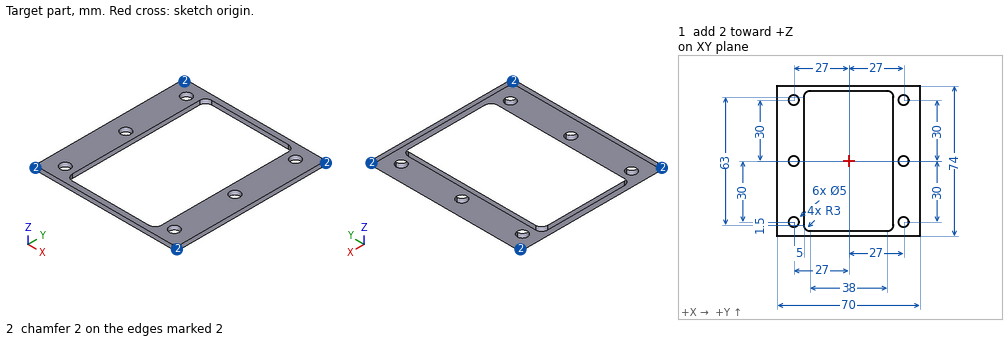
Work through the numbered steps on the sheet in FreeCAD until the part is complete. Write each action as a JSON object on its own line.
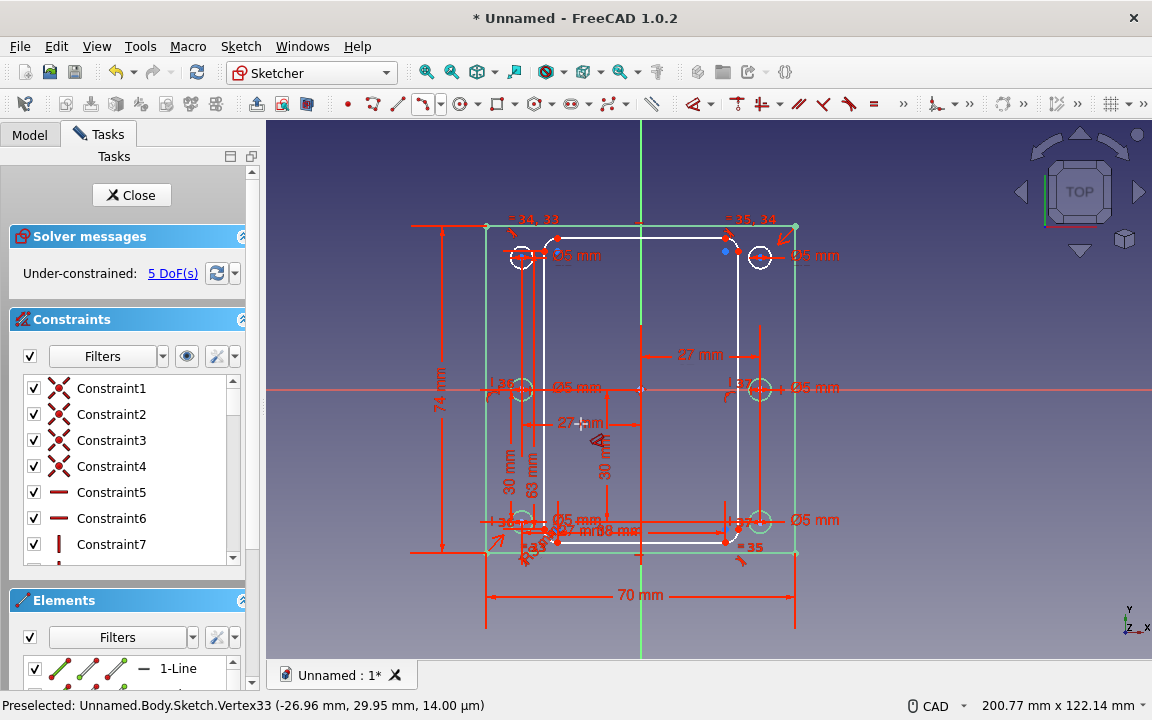
{"action": "left_click", "coordinate": [522, 258]}
{"action": "left_click", "coordinate": [675, 324]}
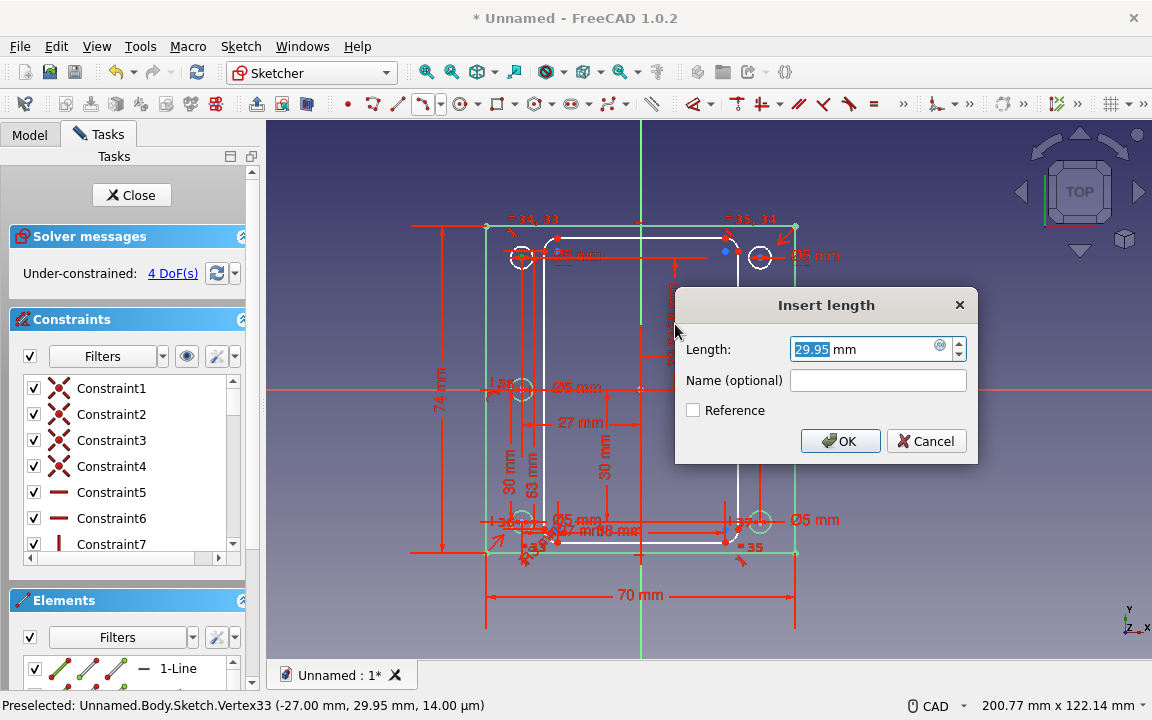
{"action": "type", "text": "30"}
{"action": "key", "text": "Return"}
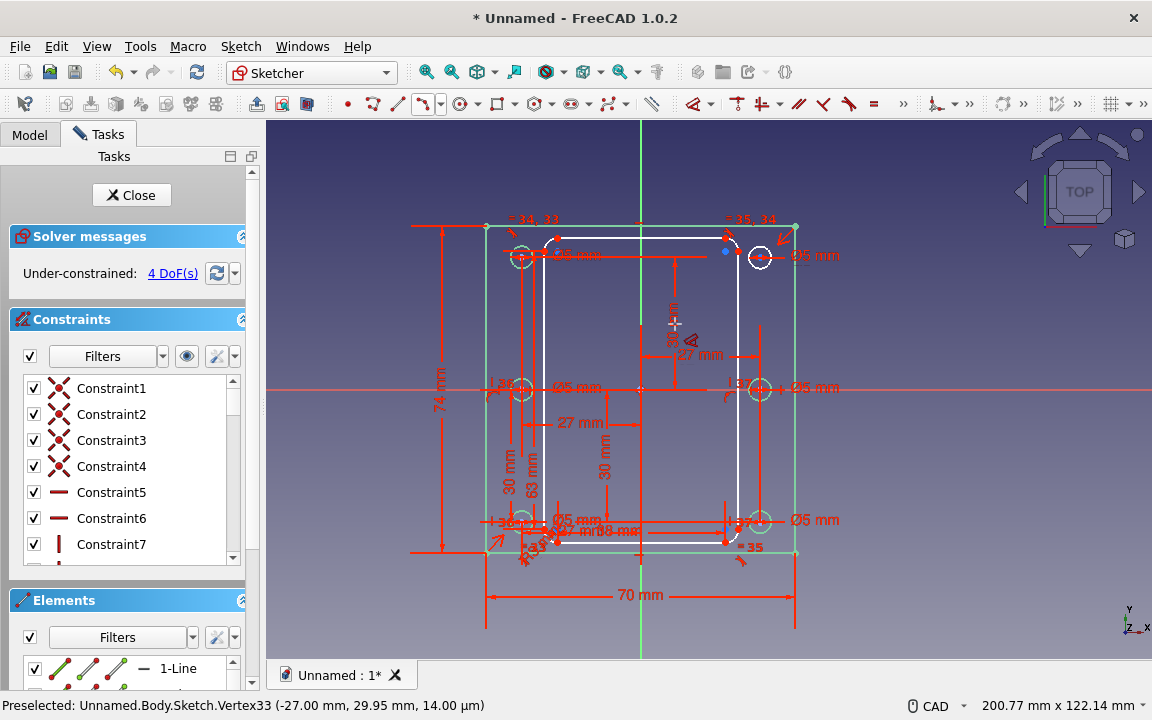
{"action": "left_click", "coordinate": [760, 258]}
{"action": "left_click", "coordinate": [701, 424]}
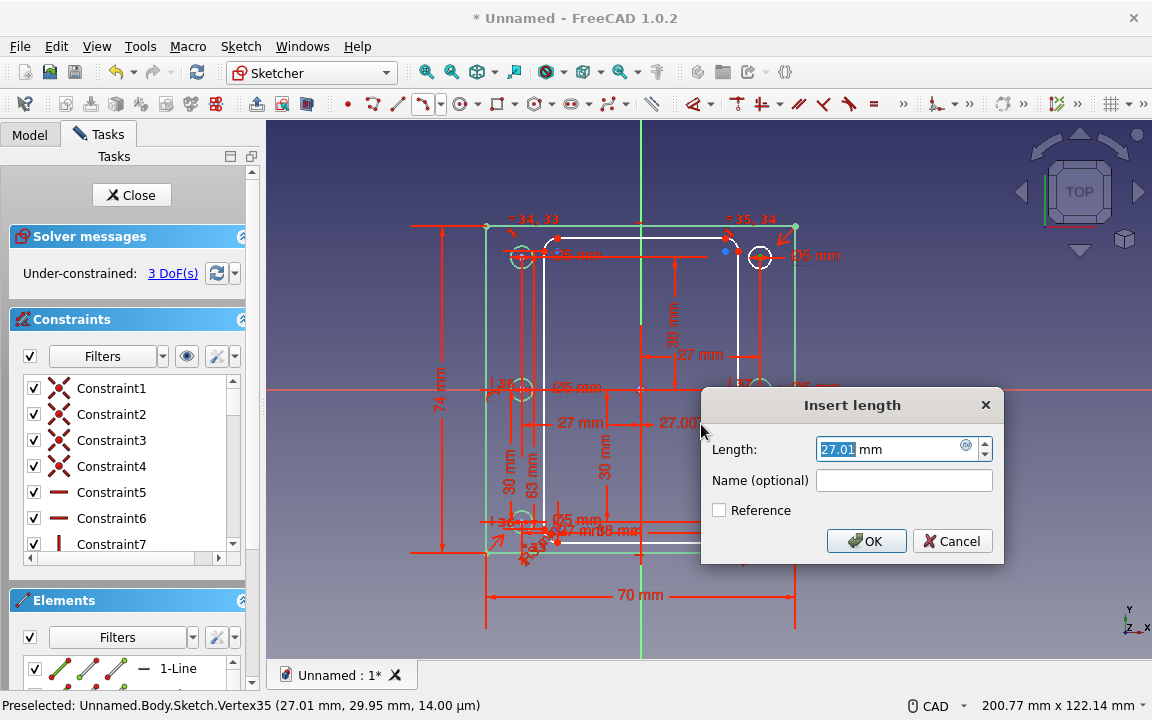
{"action": "type", "text": "27"}
{"action": "key", "text": "Return"}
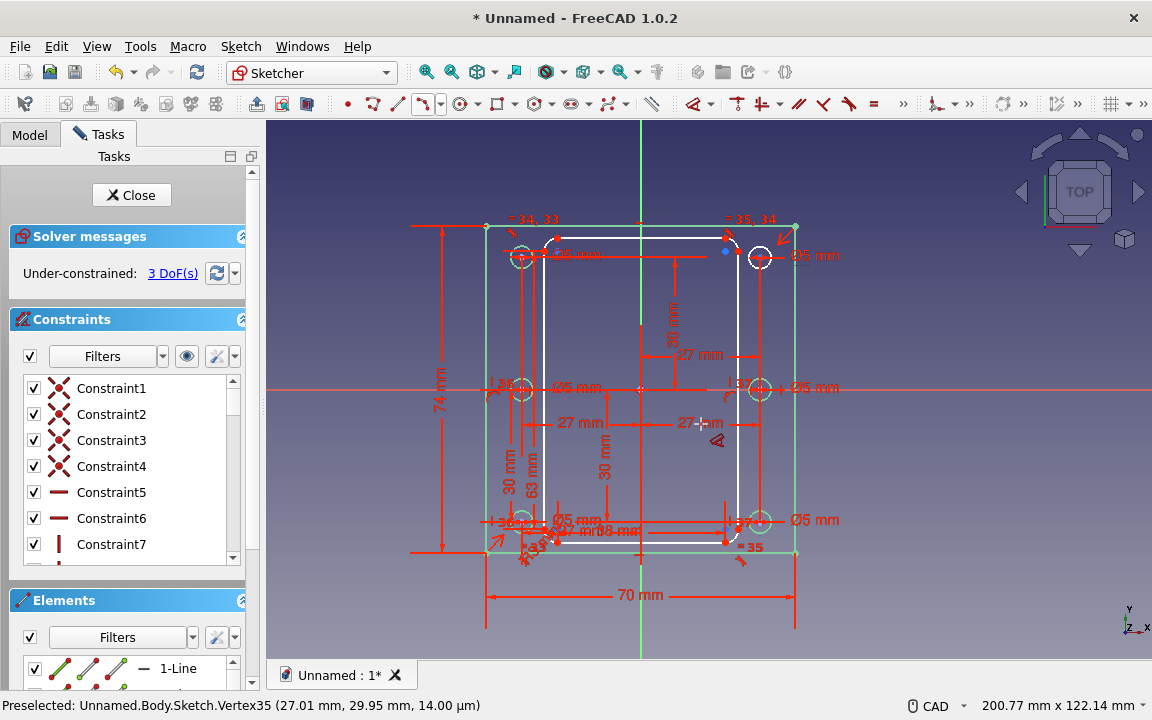
{"action": "left_click", "coordinate": [760, 258]}
{"action": "left_click", "coordinate": [607, 293]}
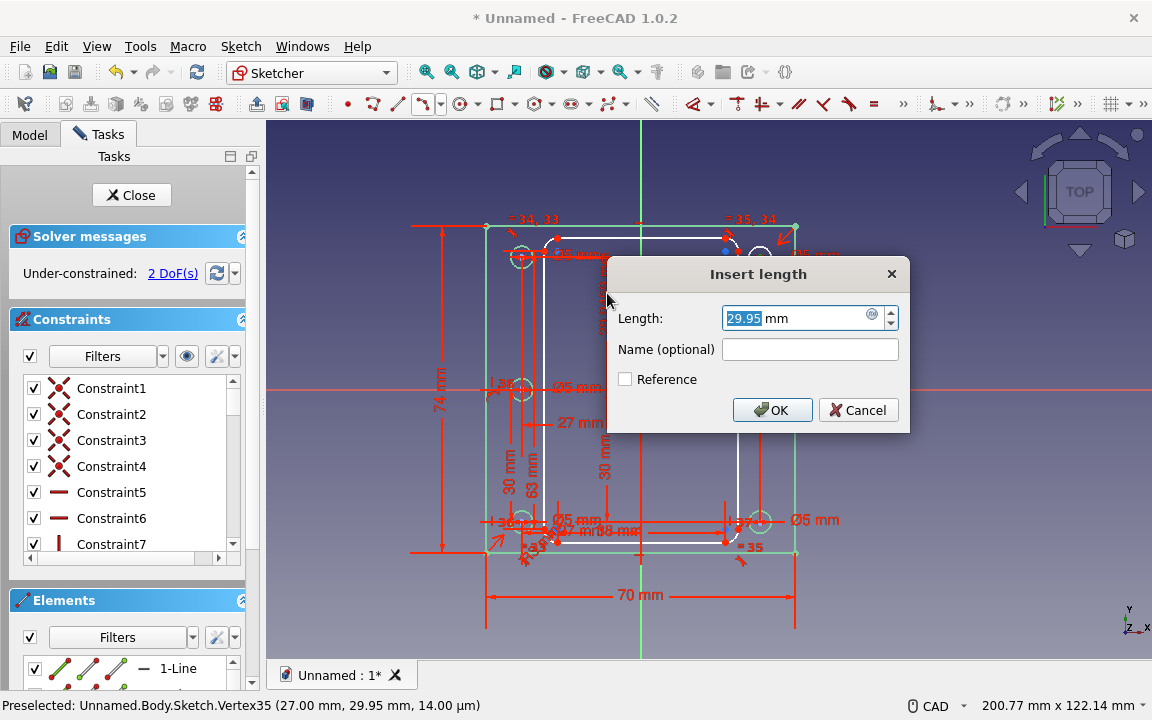
{"action": "type", "text": "30"}
{"action": "key", "text": "Return"}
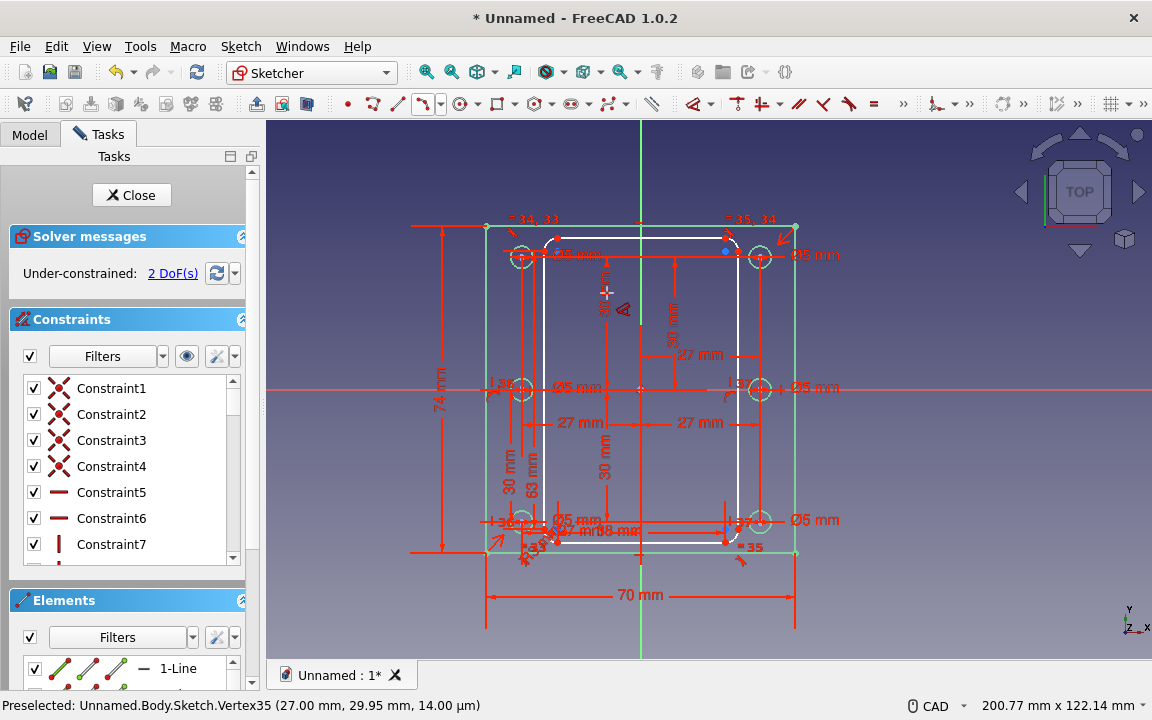
{"action": "scroll", "coordinate": [544, 529], "scroll_direction": "up", "scroll_amount": 3}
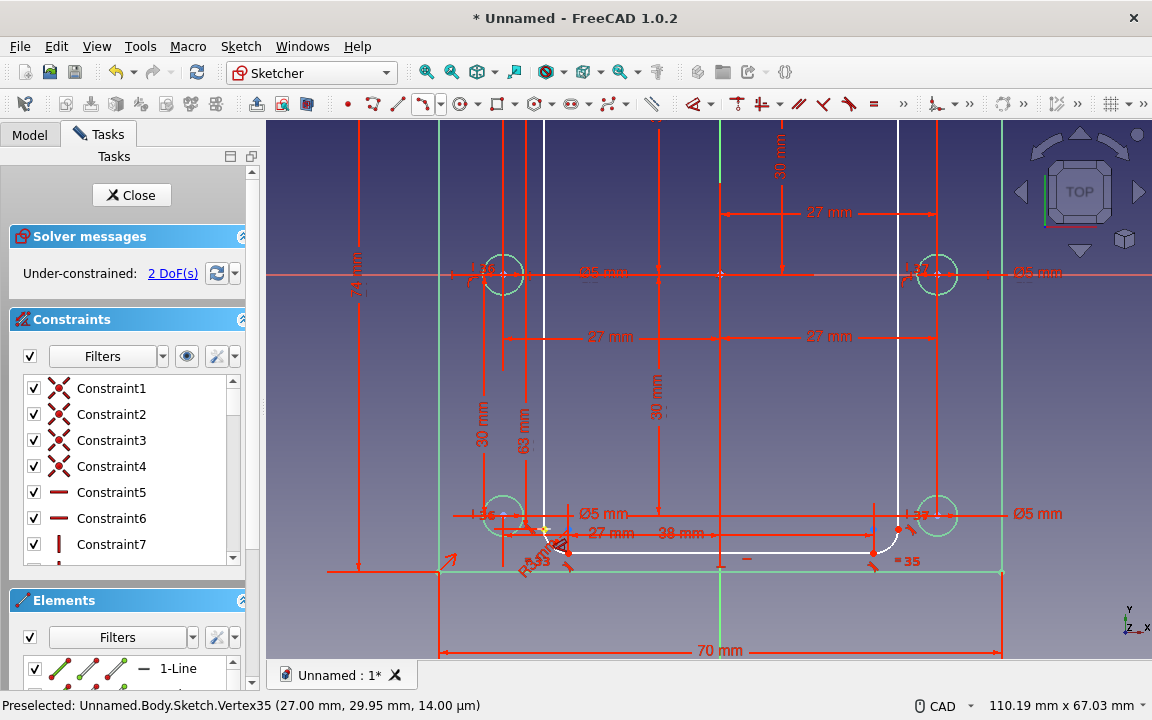
{"action": "left_click", "coordinate": [544, 529]}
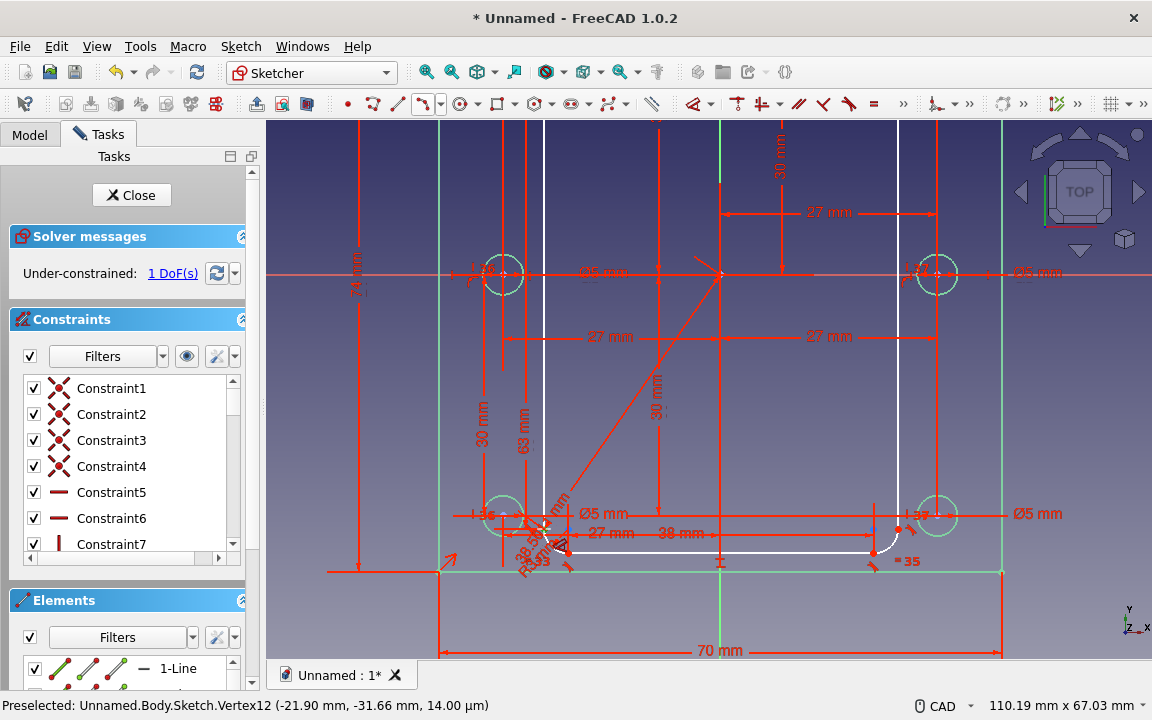
{"action": "left_click", "coordinate": [503, 516]}
{"action": "left_click", "coordinate": [524, 482]}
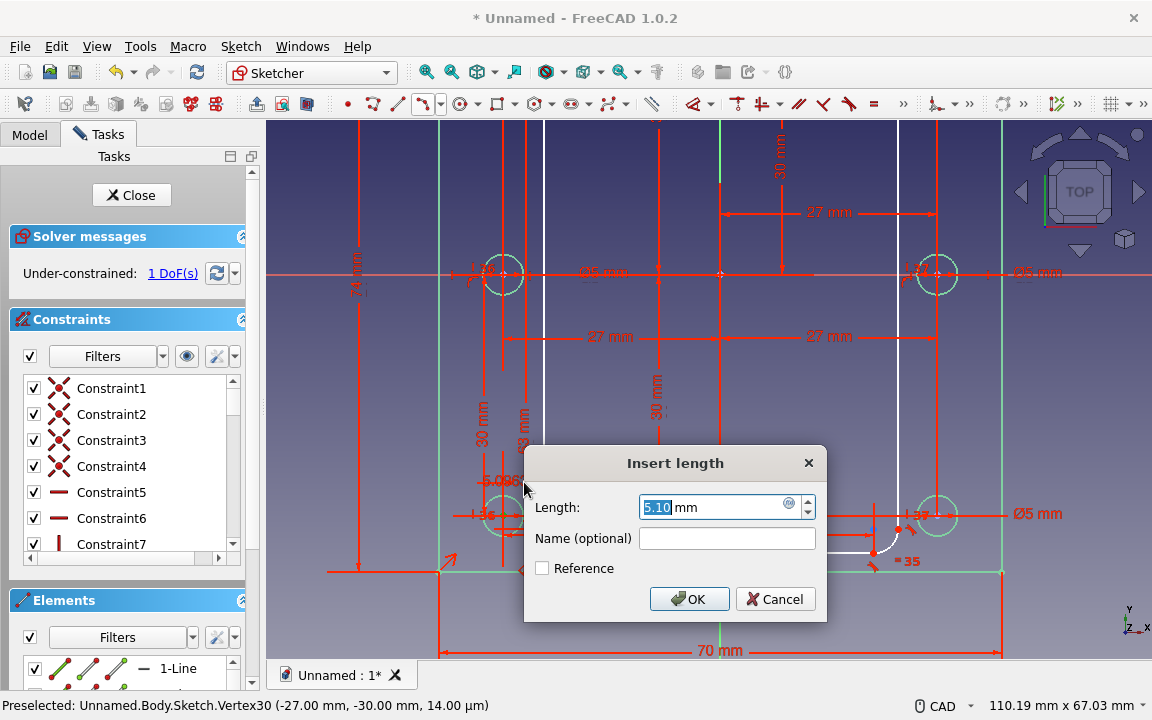
{"action": "type", "text": "5"}
{"action": "key", "text": "Return"}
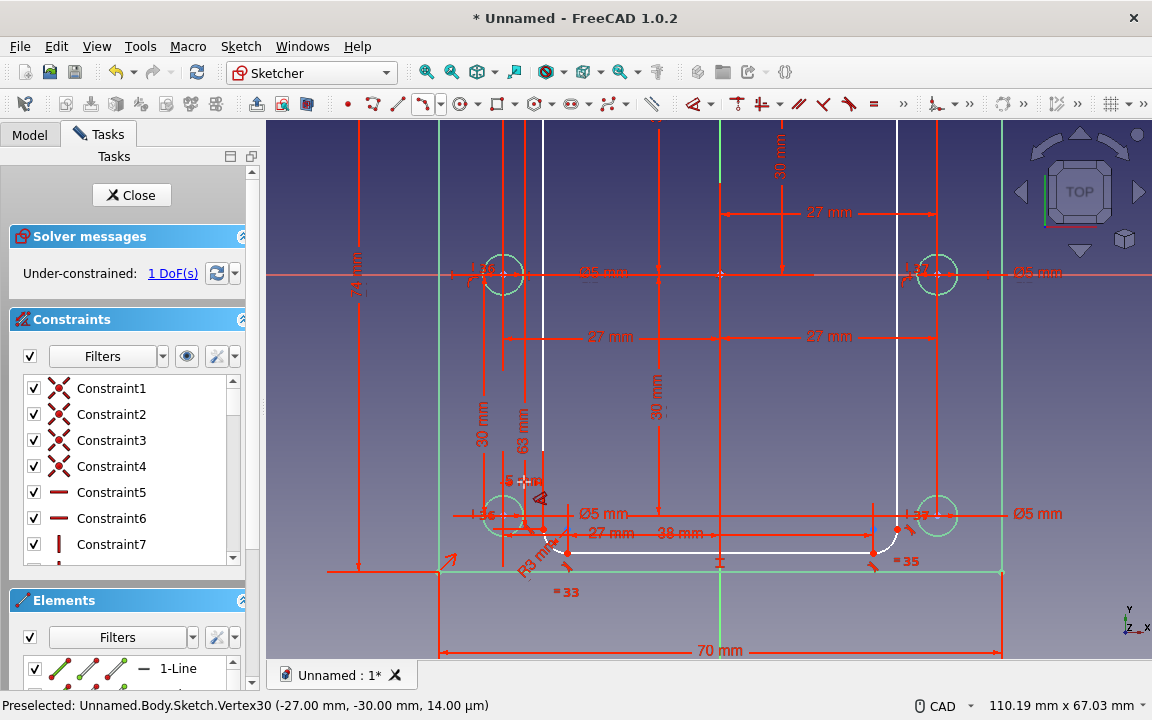
{"action": "scroll", "coordinate": [543, 529], "scroll_direction": "up", "scroll_amount": 6}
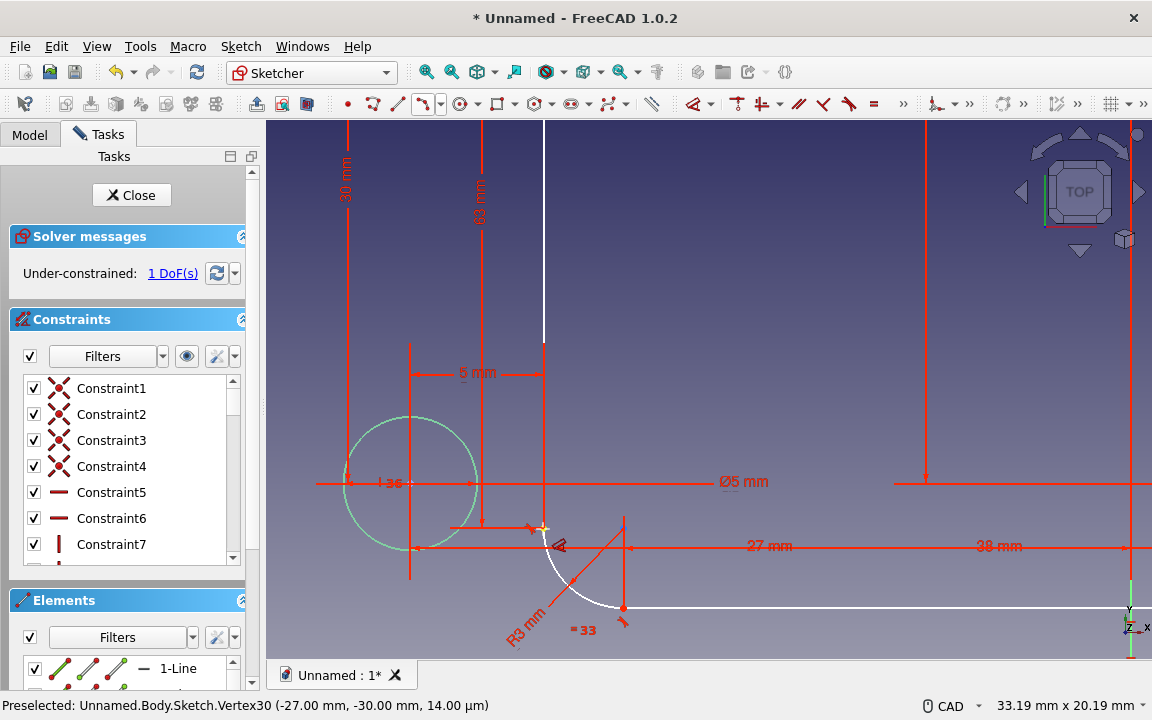
{"action": "left_click", "coordinate": [544, 528]}